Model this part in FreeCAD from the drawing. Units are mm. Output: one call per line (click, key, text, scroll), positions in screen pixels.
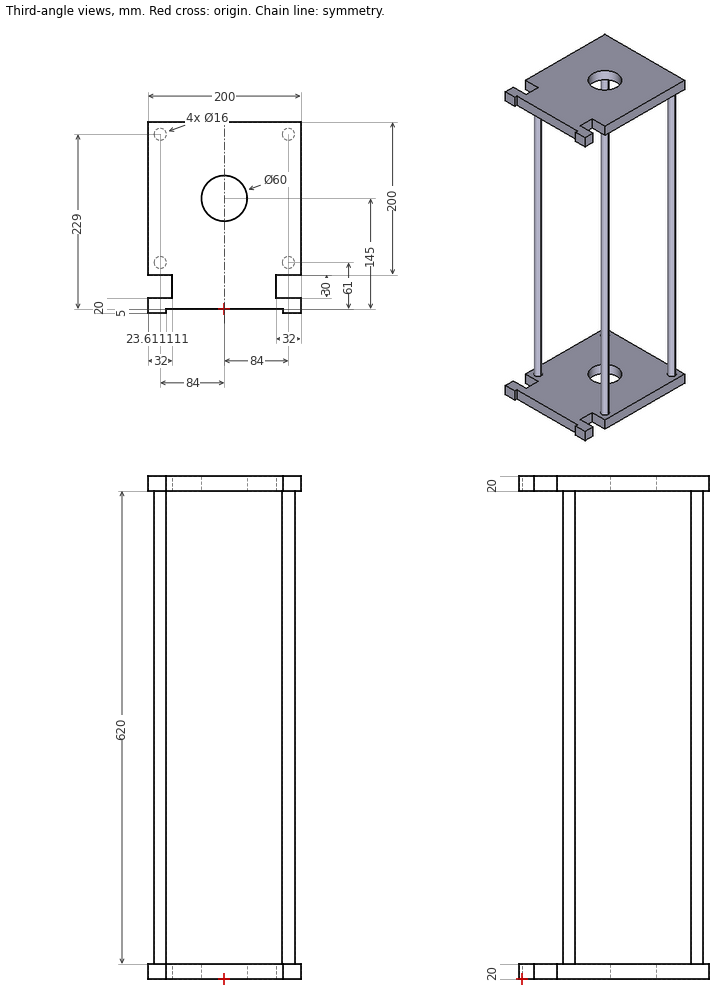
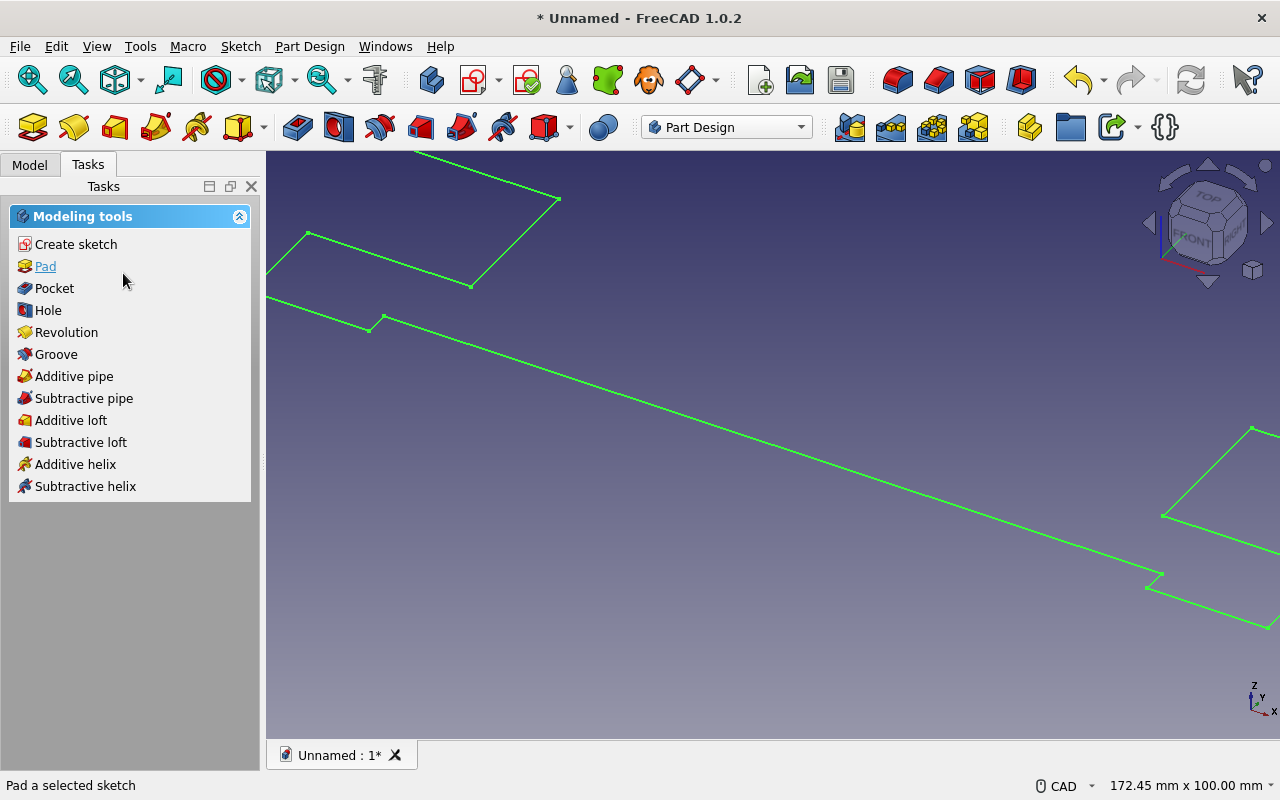
click(33, 128)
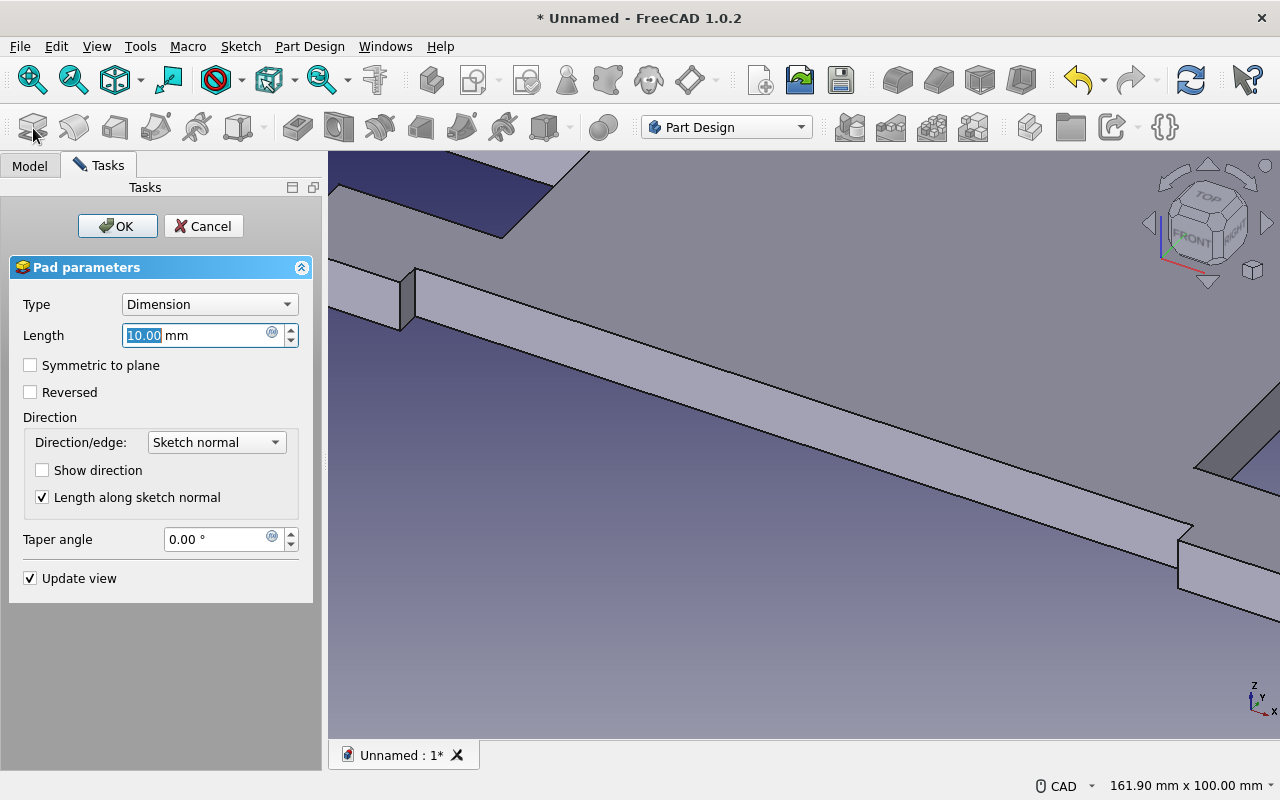
text(20)
key(Tab)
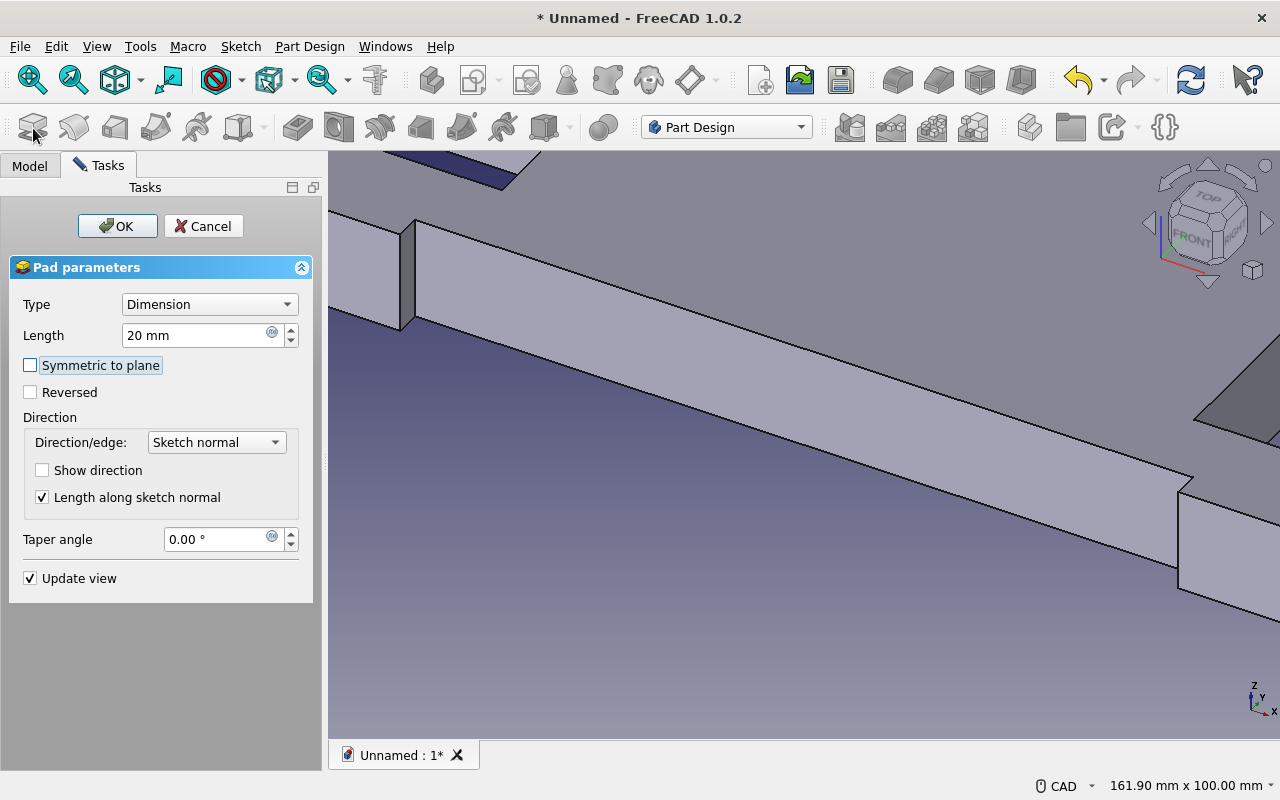
click(118, 226)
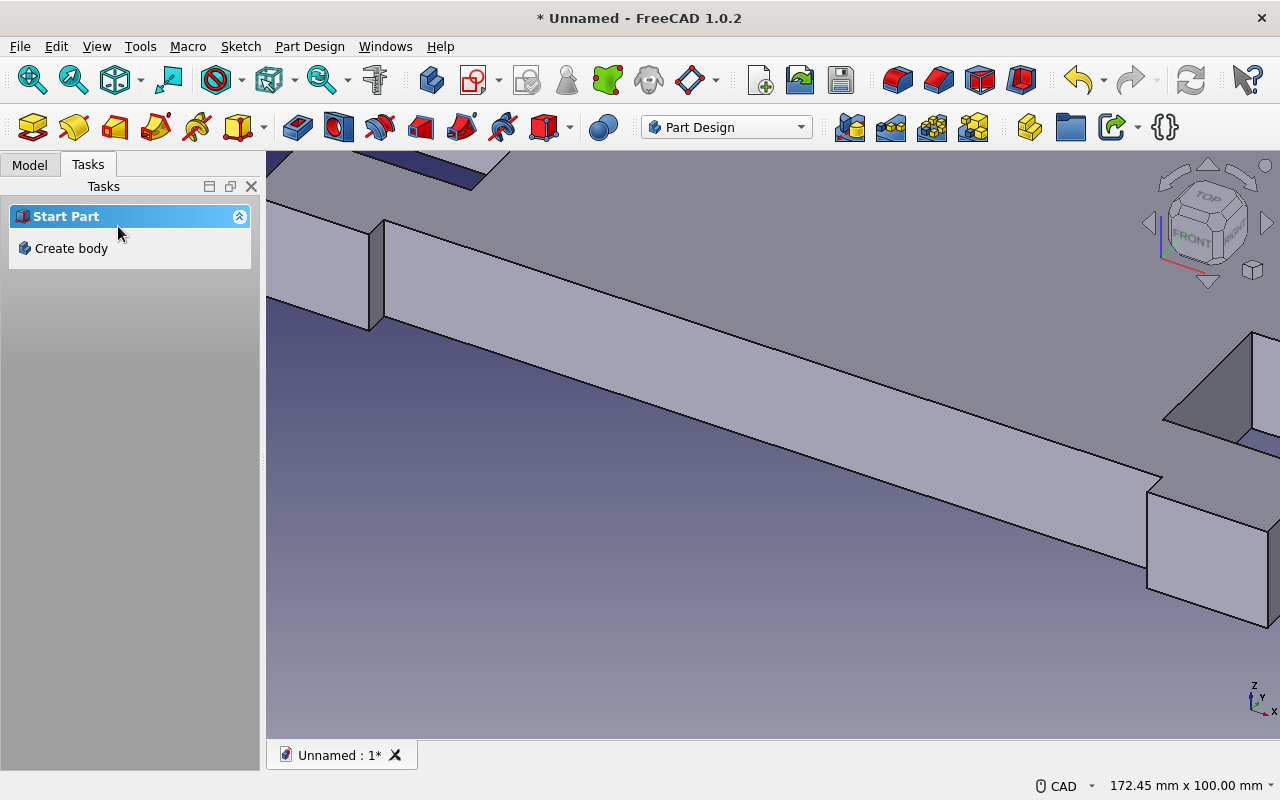
click(33, 80)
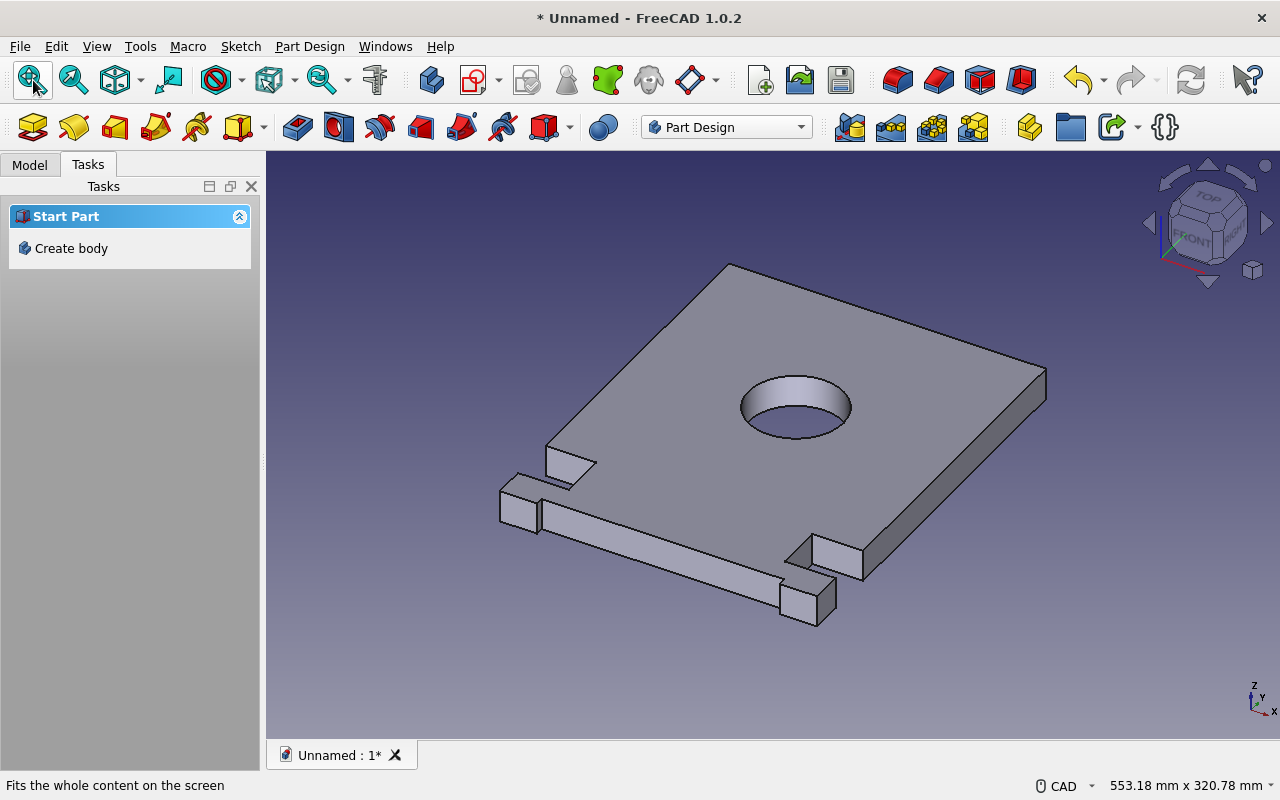
click(708, 494)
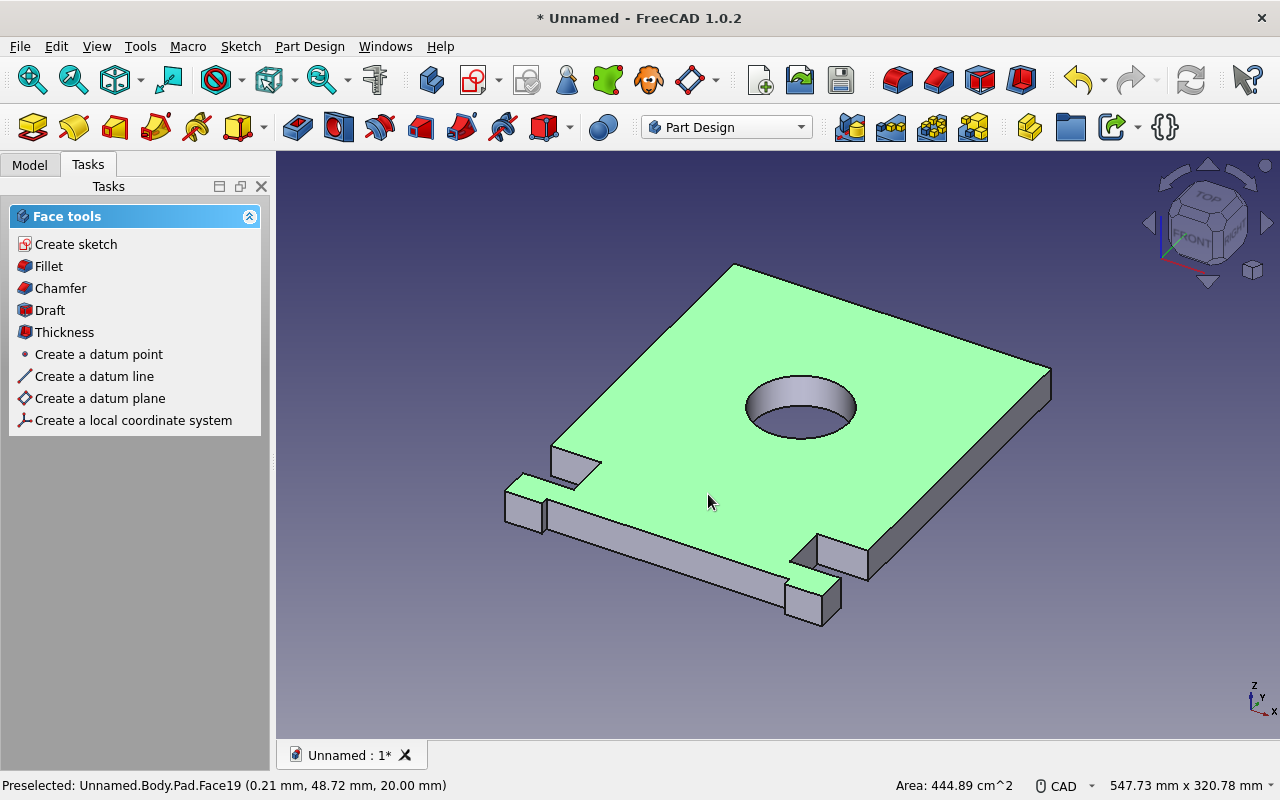
click(472, 80)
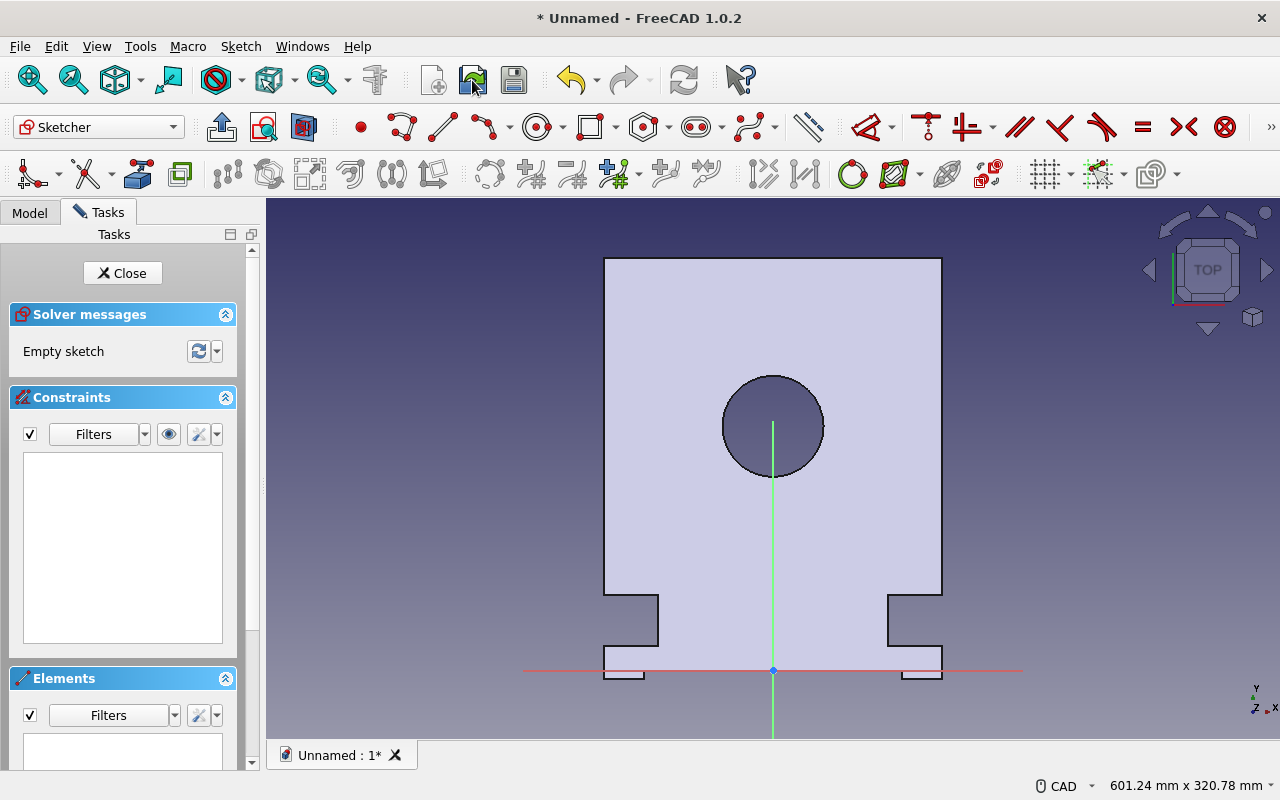
click(536, 128)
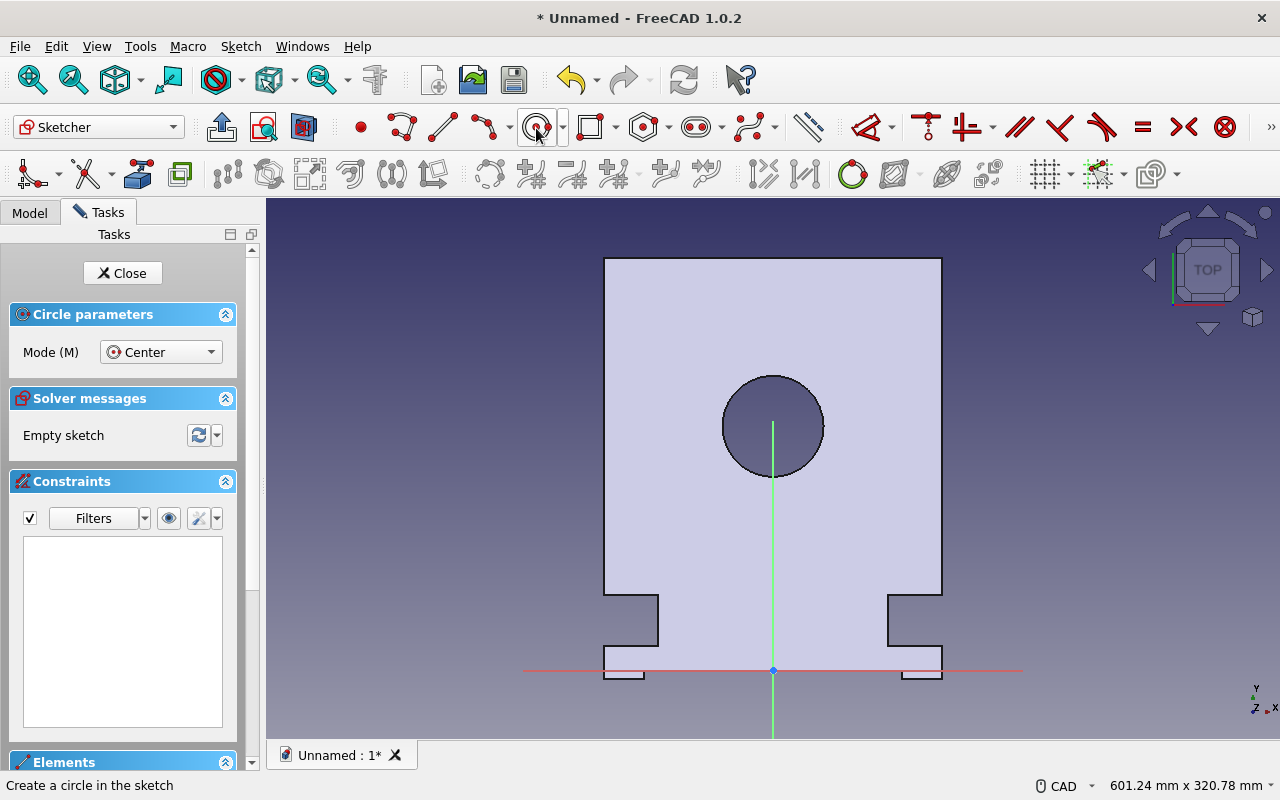
scroll(631, 285, up, 3)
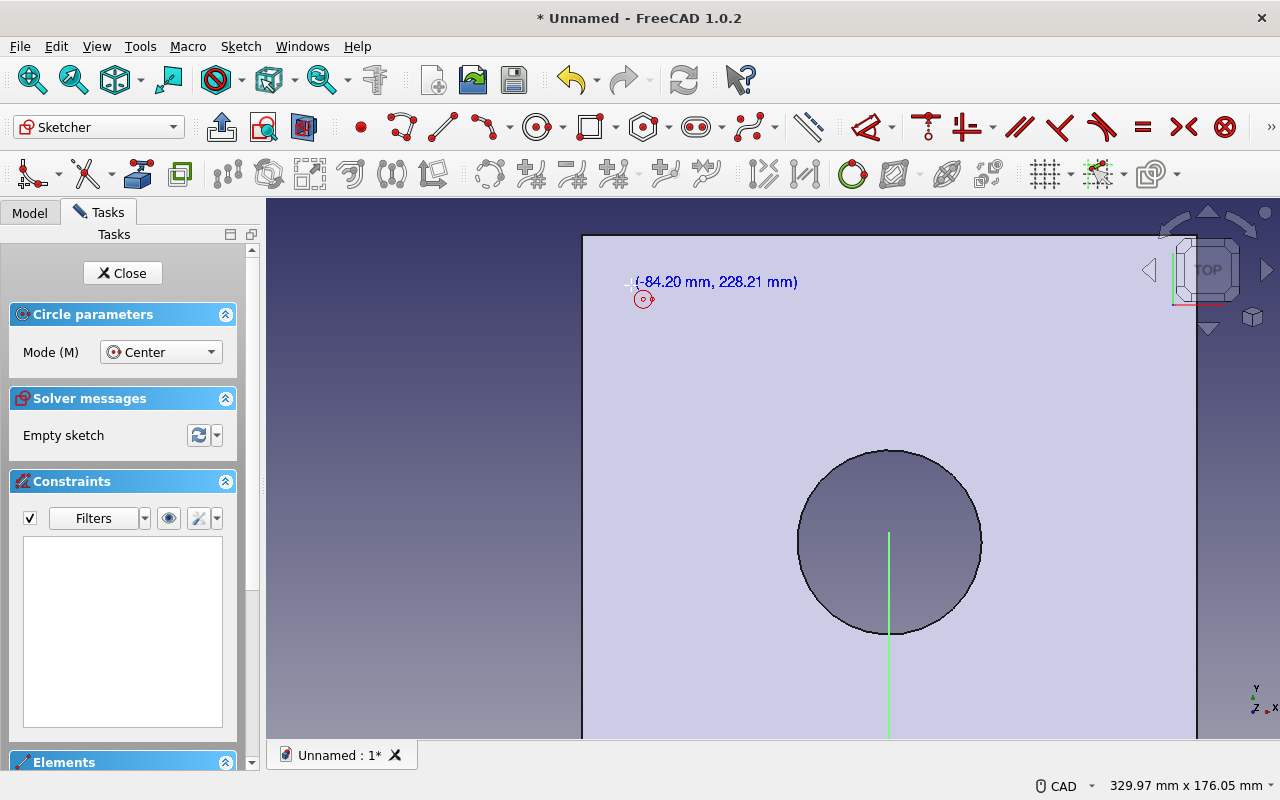
click(631, 284)
click(649, 267)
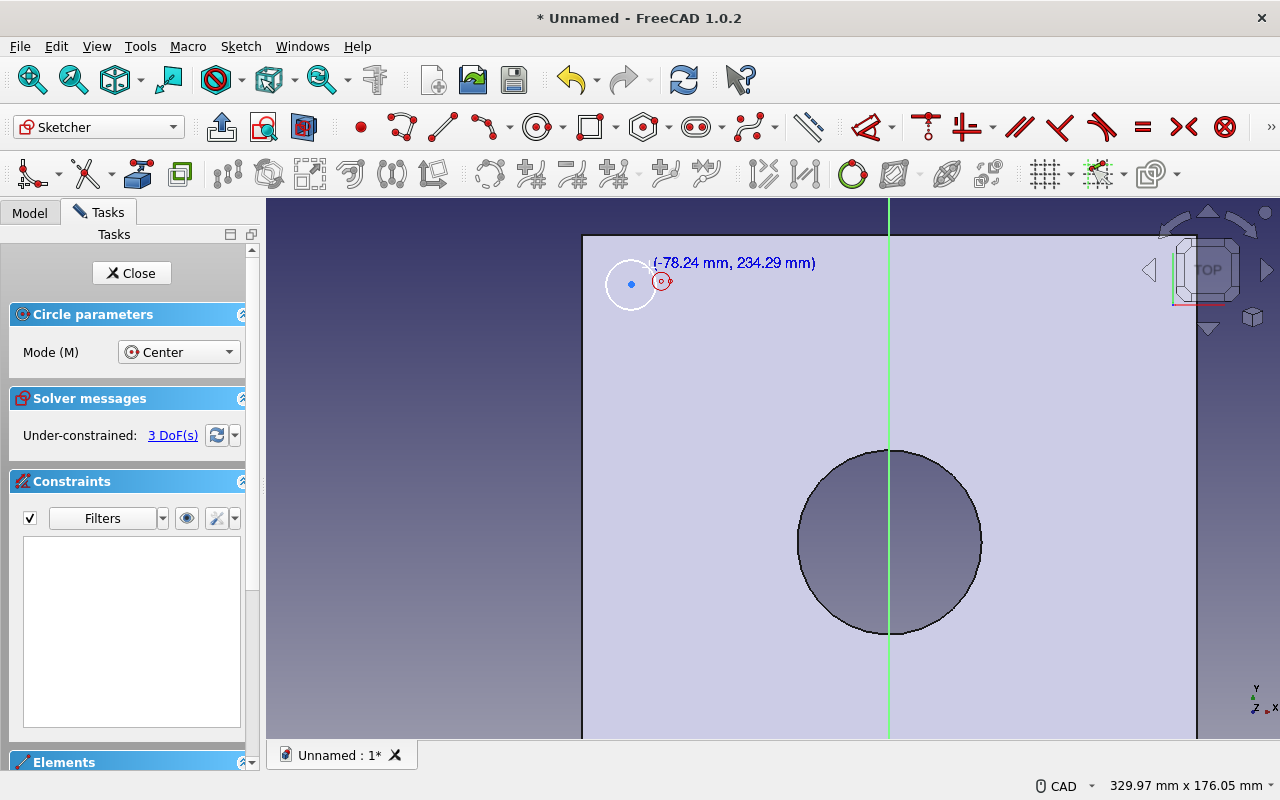
scroll(554, 342, down, 4)